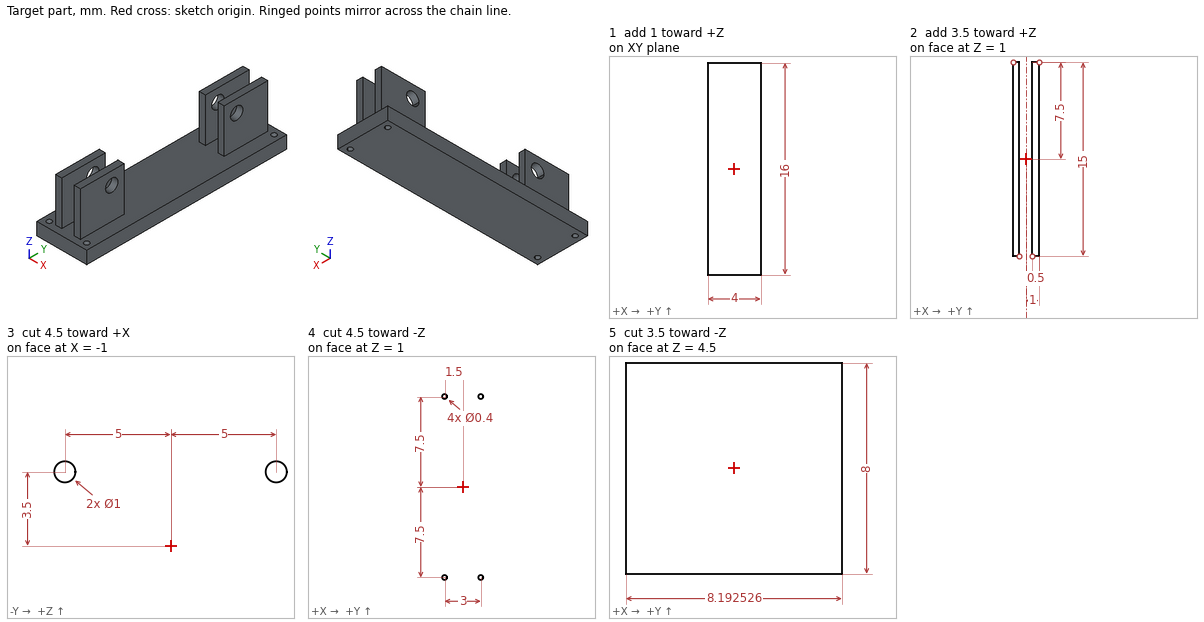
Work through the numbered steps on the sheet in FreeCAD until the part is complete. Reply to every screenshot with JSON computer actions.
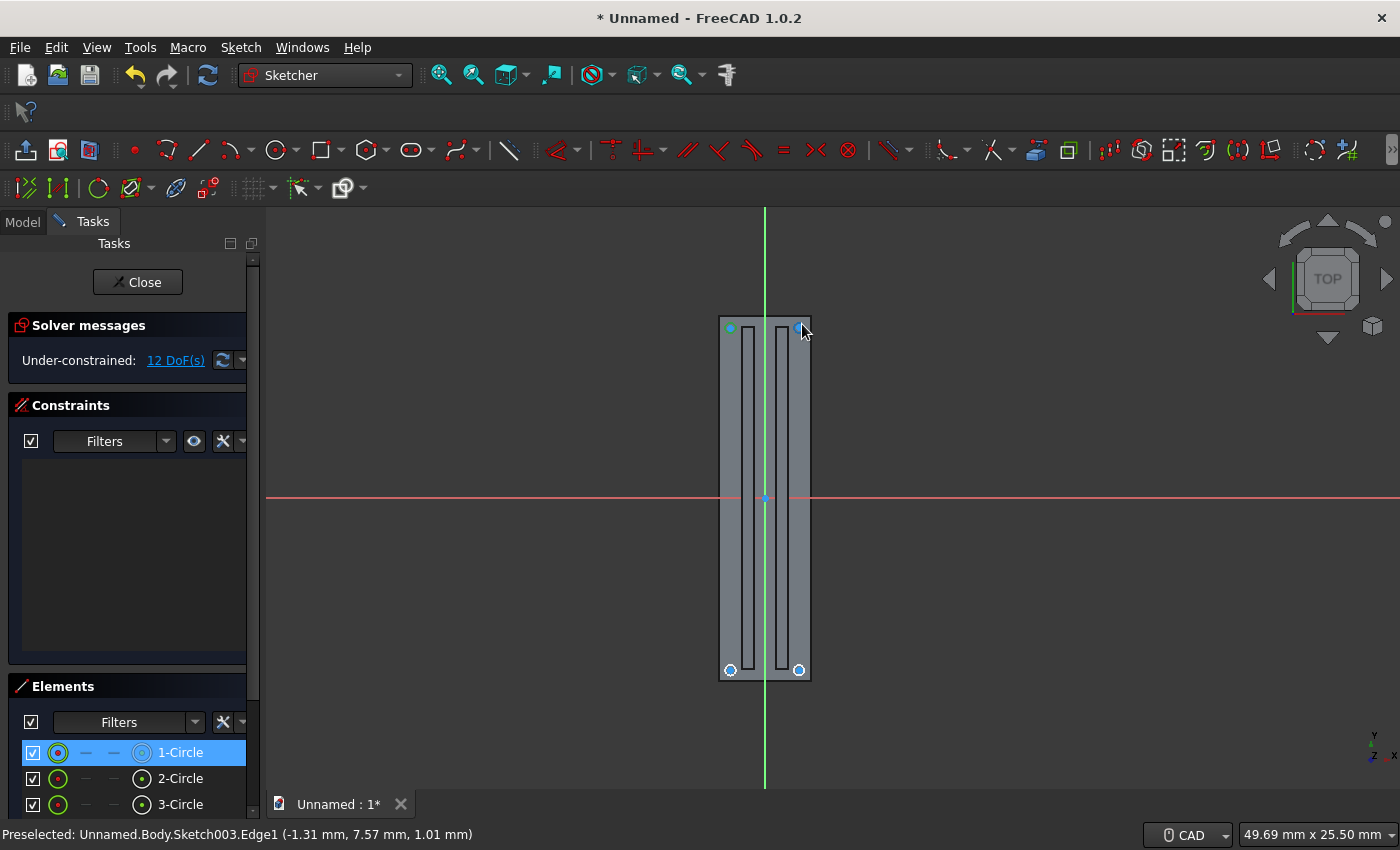
{"action": "scroll", "coordinate": [734, 667], "scroll_direction": "up", "scroll_amount": 5}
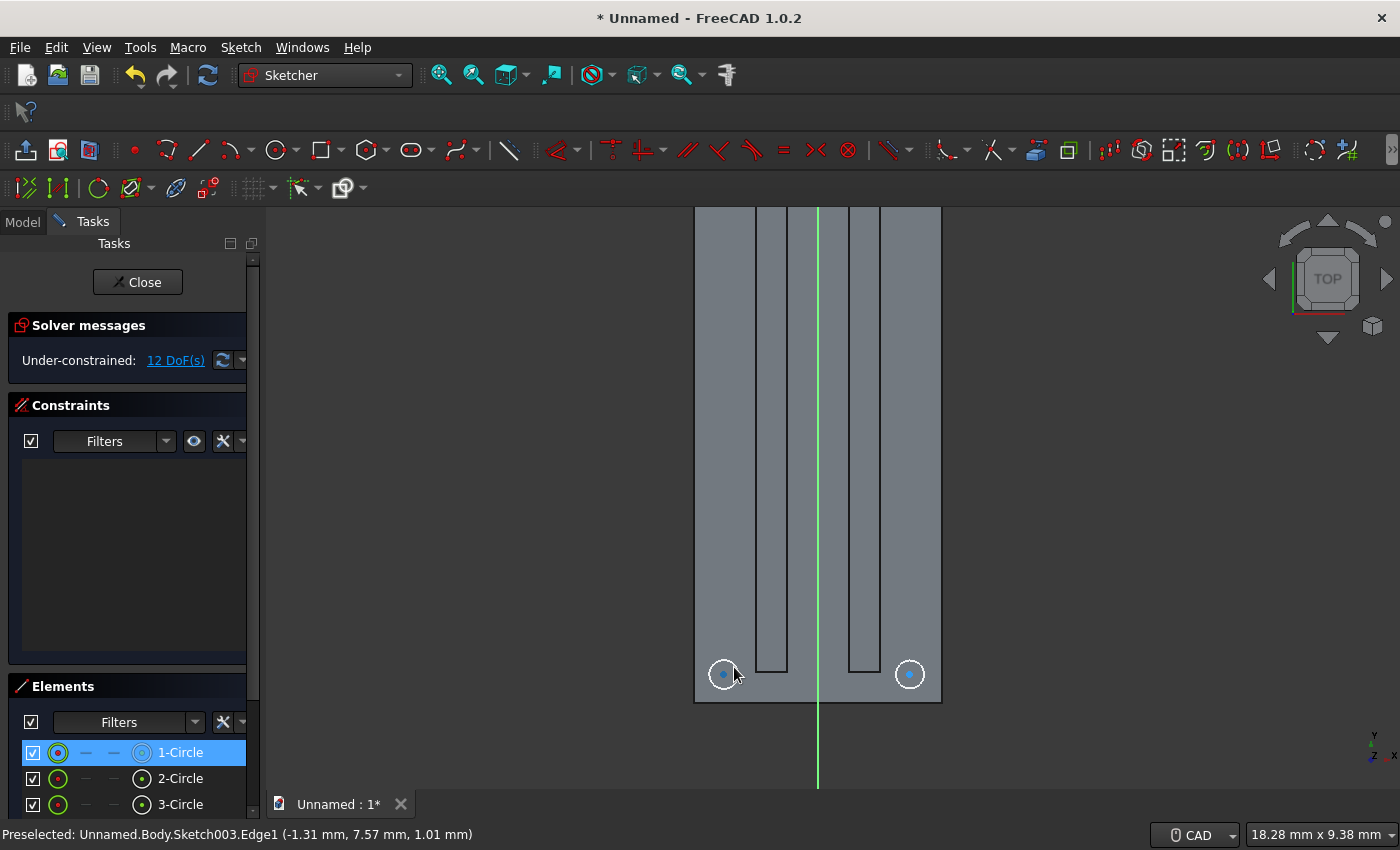
{"action": "left_click", "coordinate": [734, 664]}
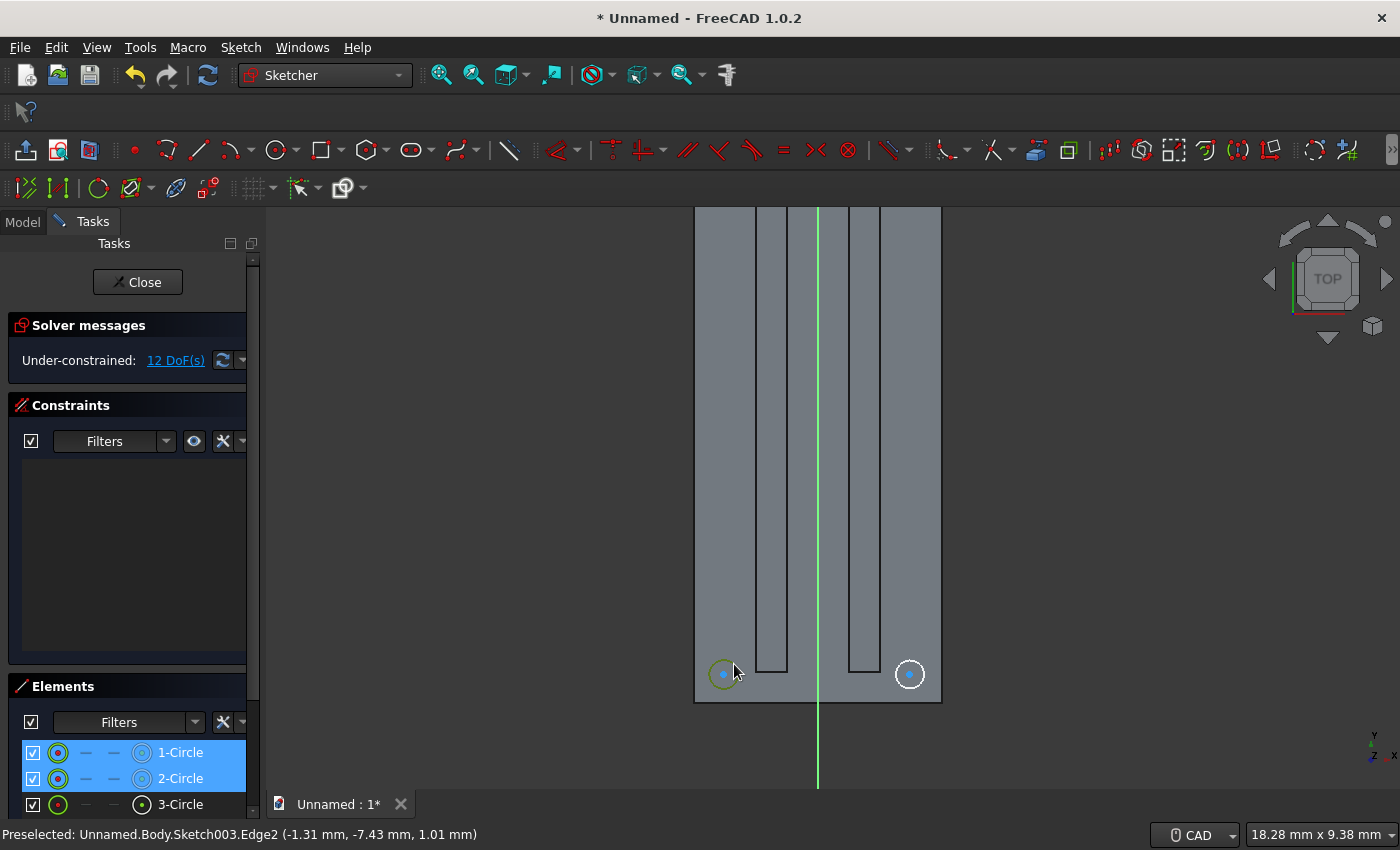
{"action": "left_click", "coordinate": [920, 665]}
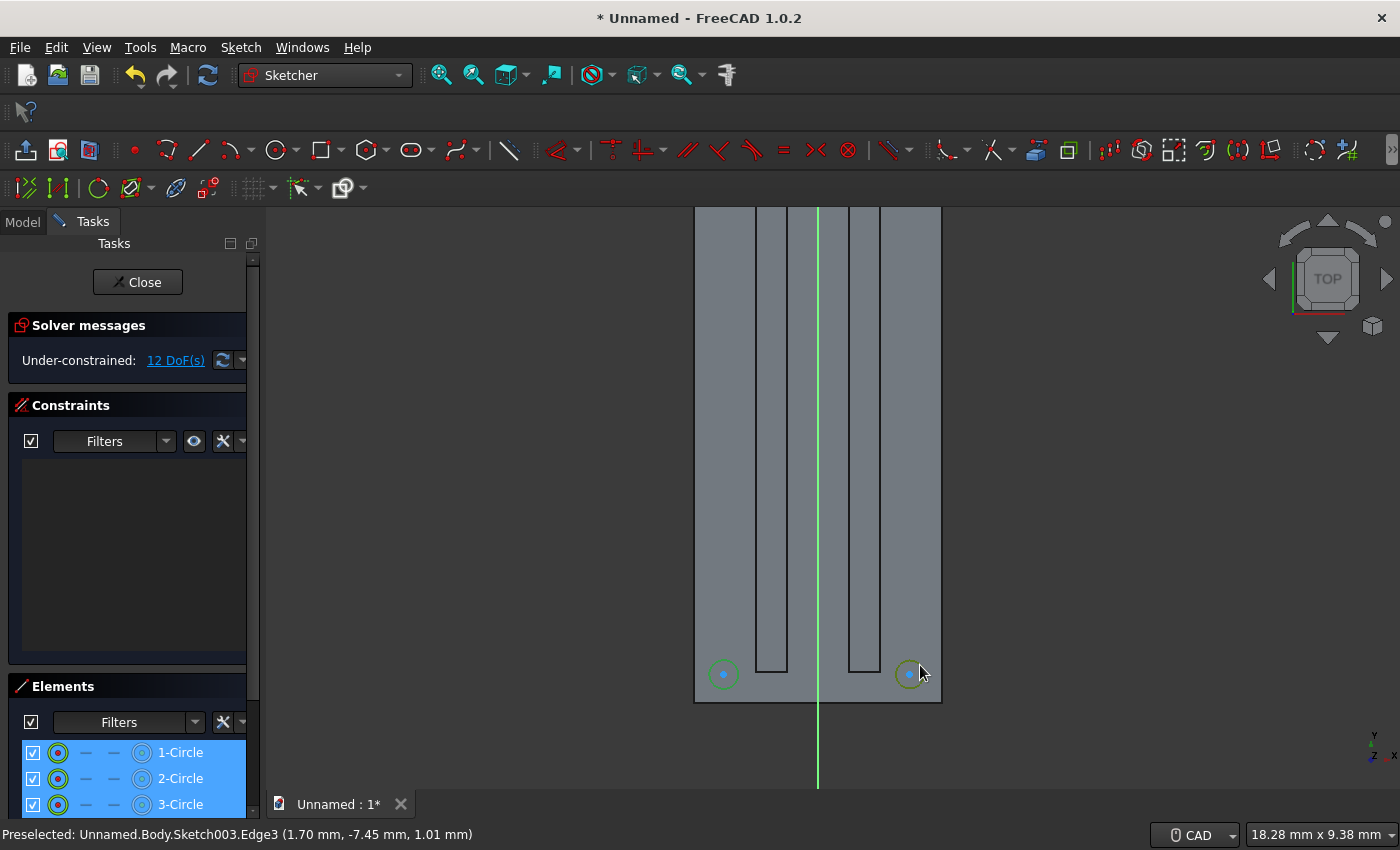
{"action": "scroll", "coordinate": [734, 667], "scroll_direction": "down", "scroll_amount": 5}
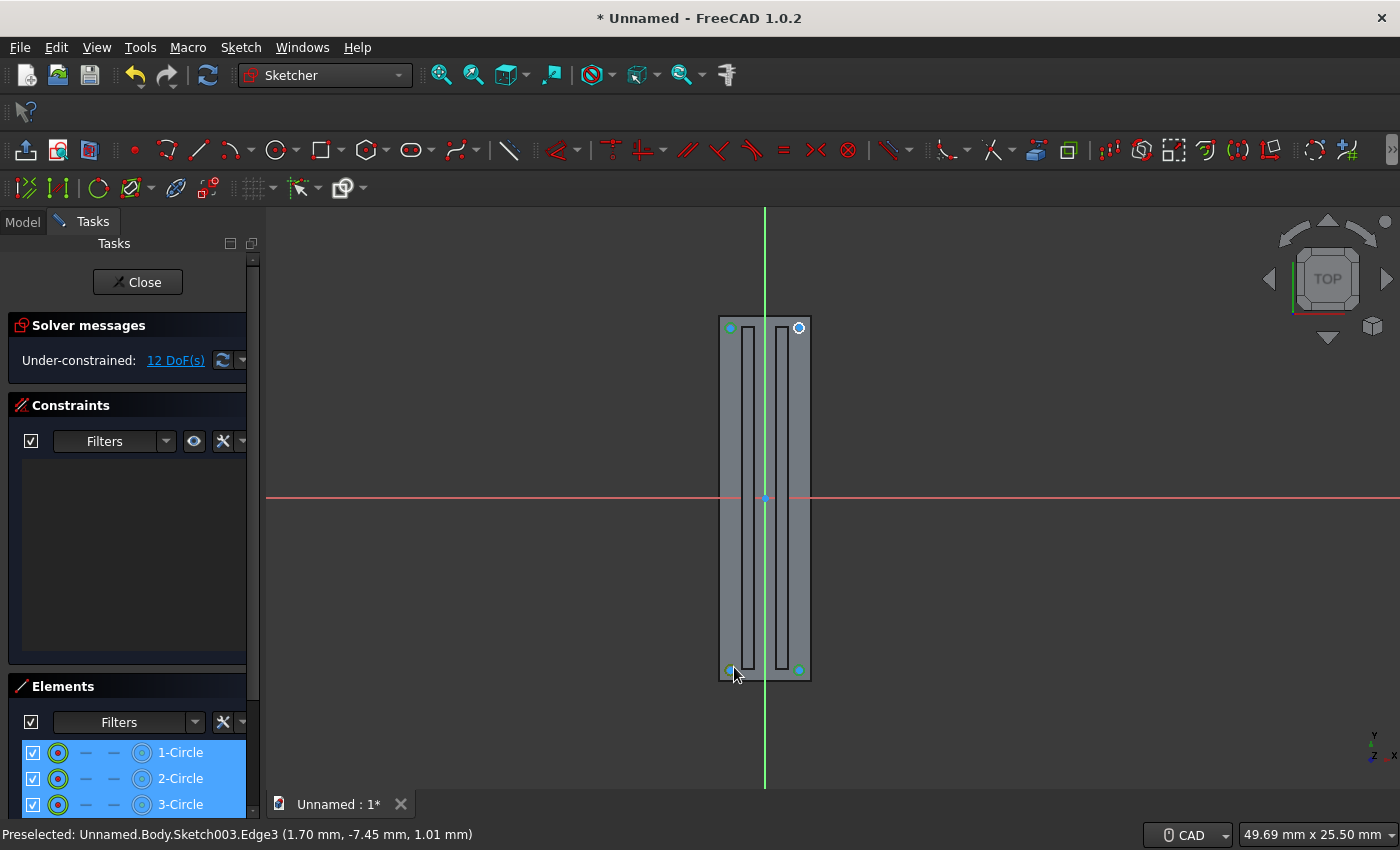
{"action": "scroll", "coordinate": [803, 324], "scroll_direction": "up", "scroll_amount": 5}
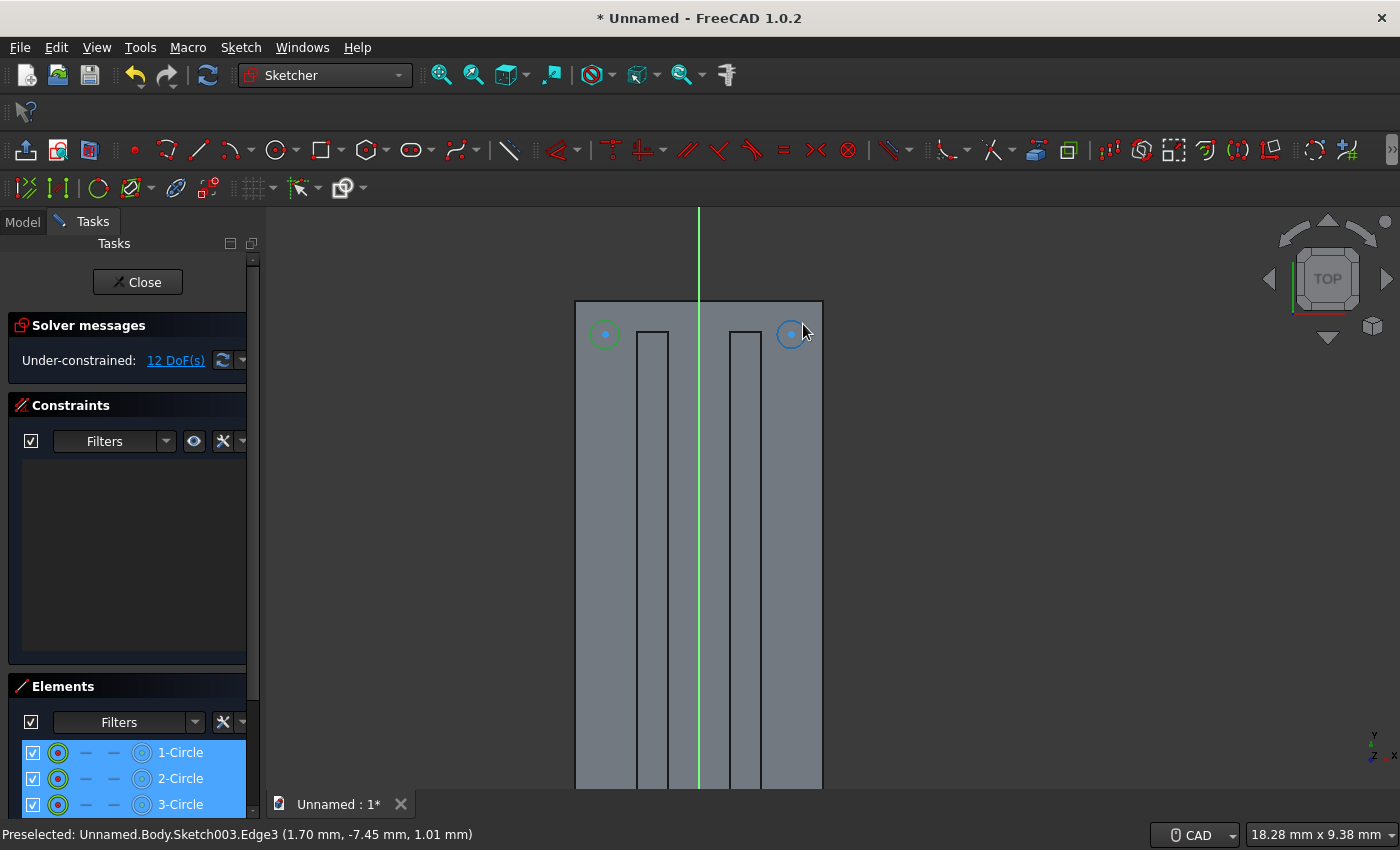
{"action": "left_click", "coordinate": [801, 325]}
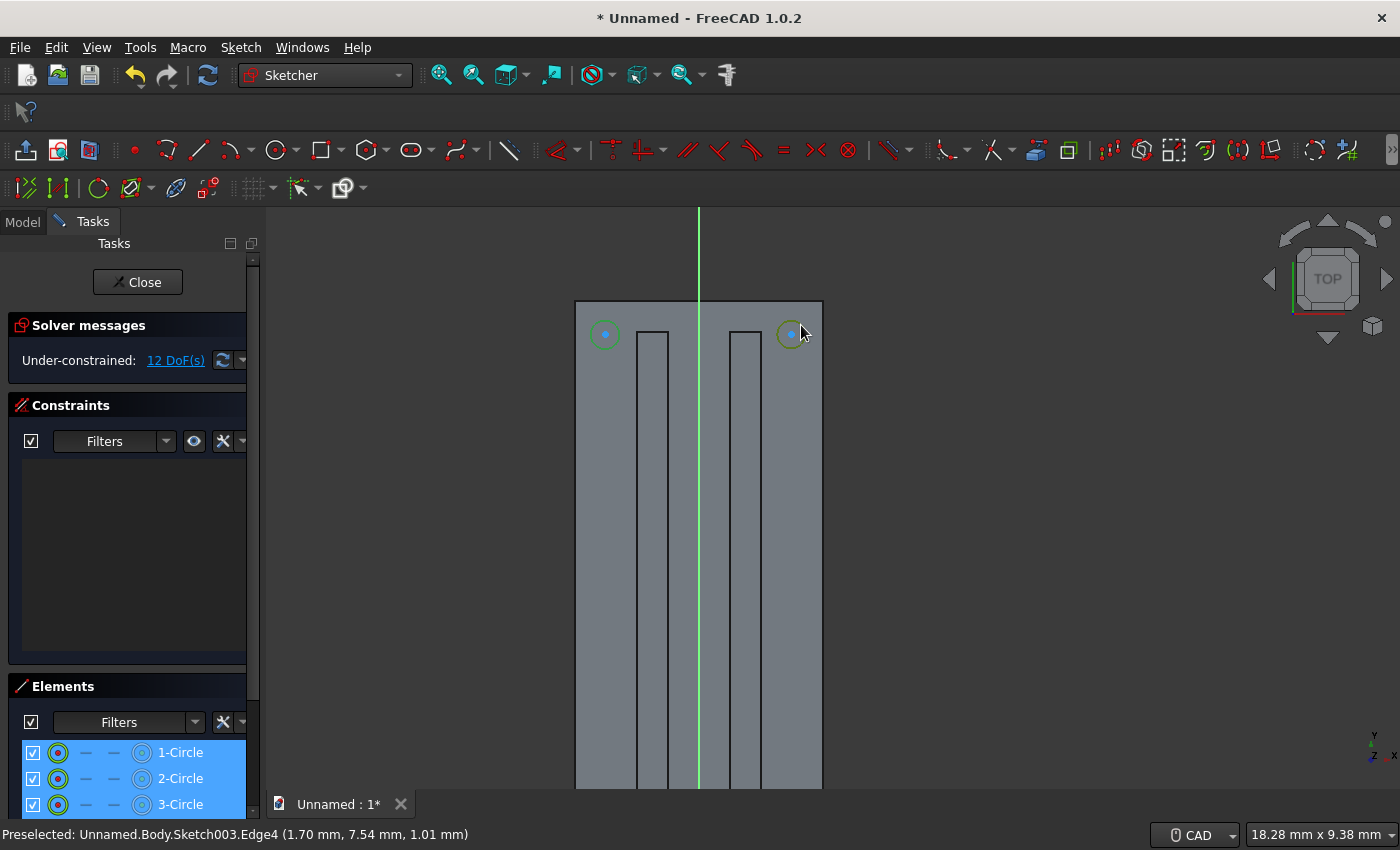
{"action": "key", "text": "e"}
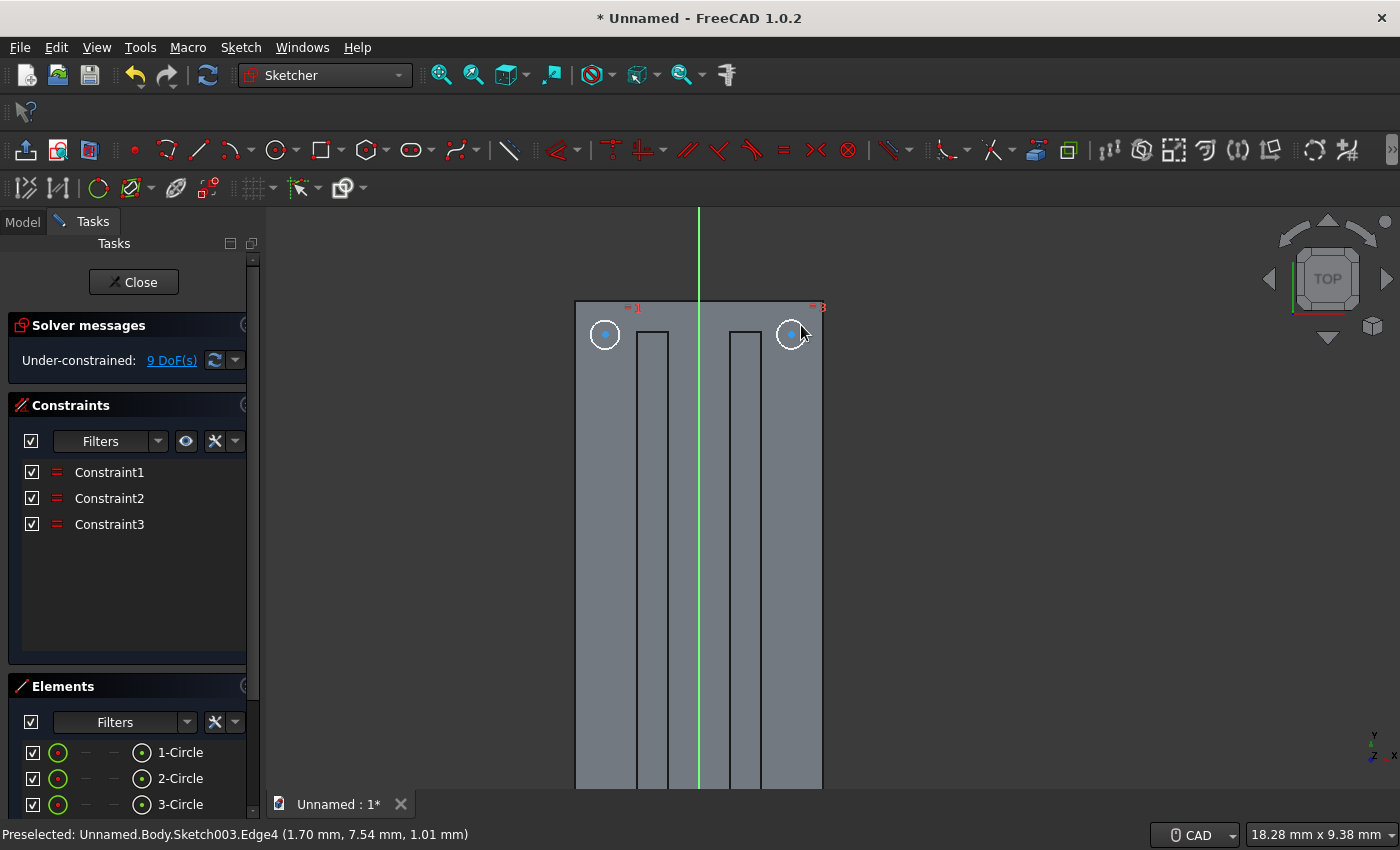
{"action": "left_click", "coordinate": [605, 335]}